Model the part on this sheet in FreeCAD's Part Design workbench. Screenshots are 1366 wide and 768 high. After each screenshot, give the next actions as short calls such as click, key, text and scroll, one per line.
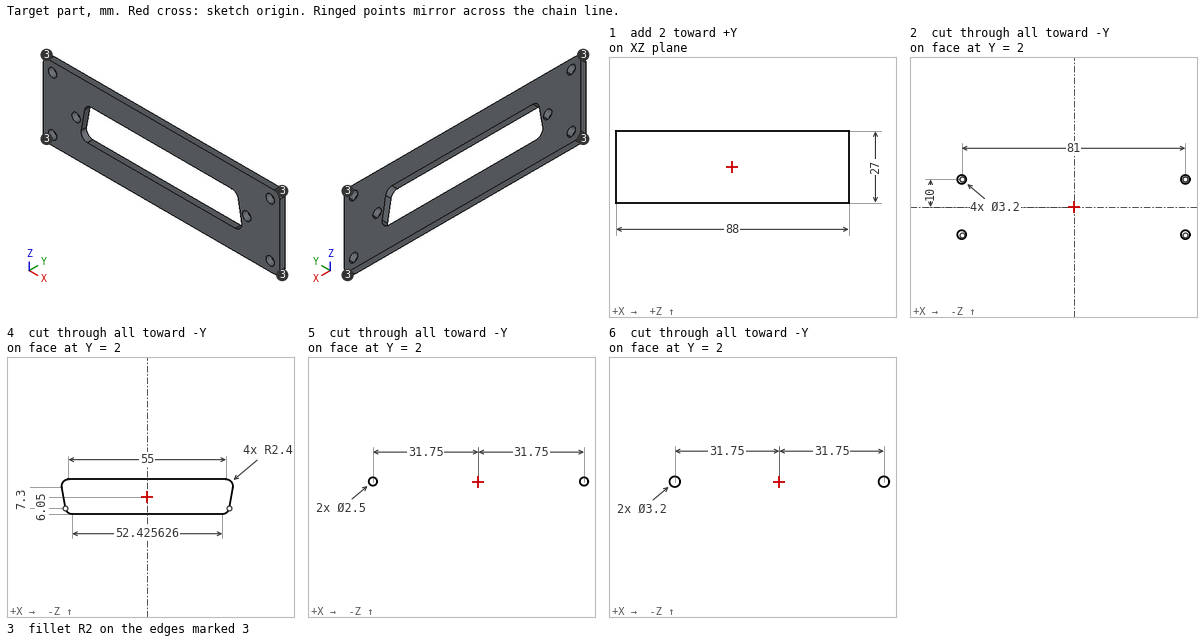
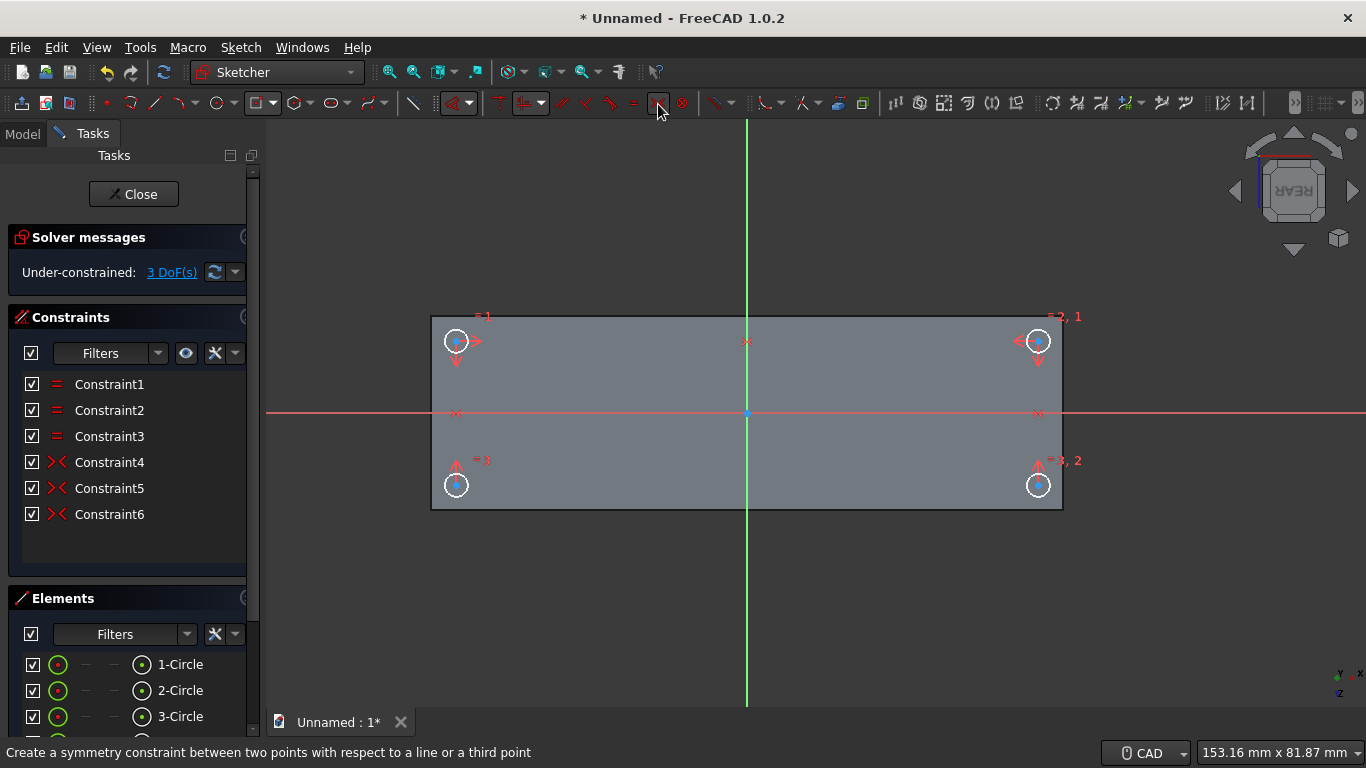
scroll(464, 333, up, 3)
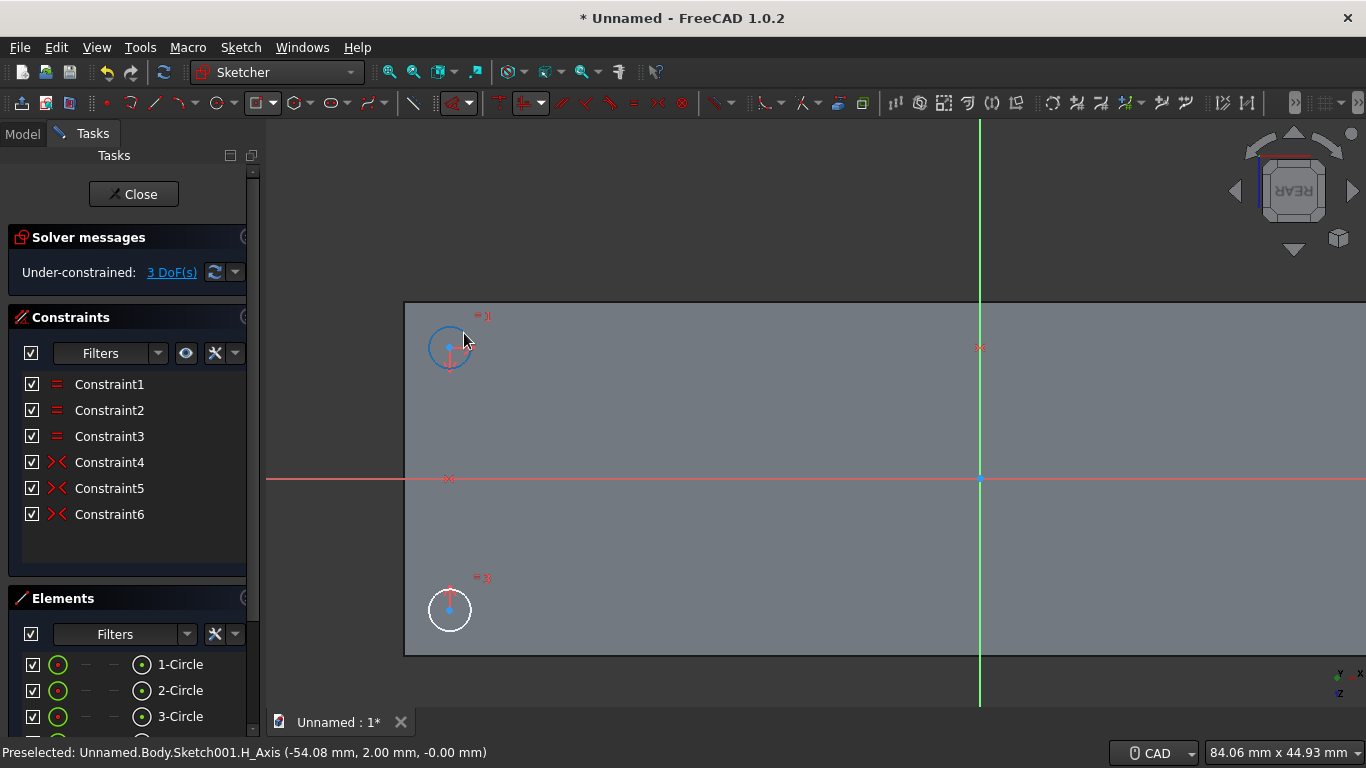
click(465, 333)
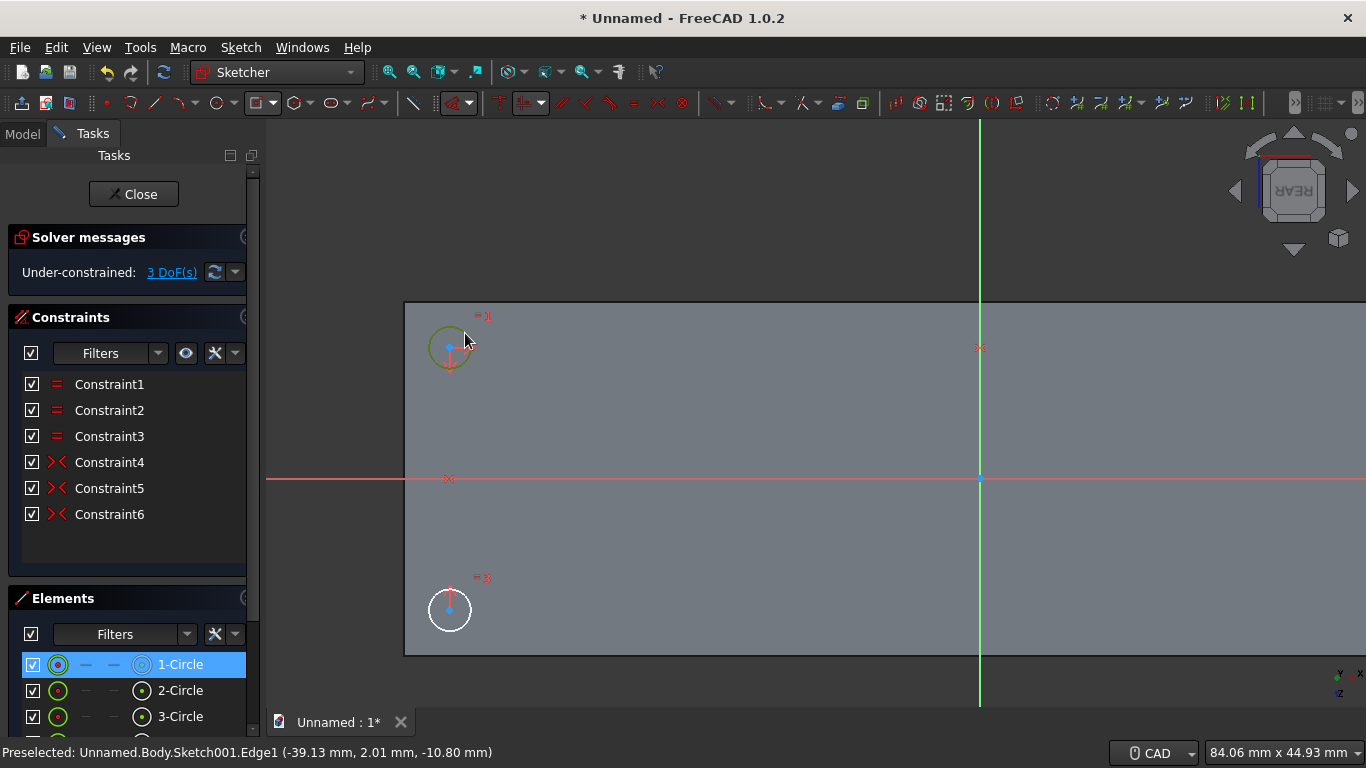
click(472, 104)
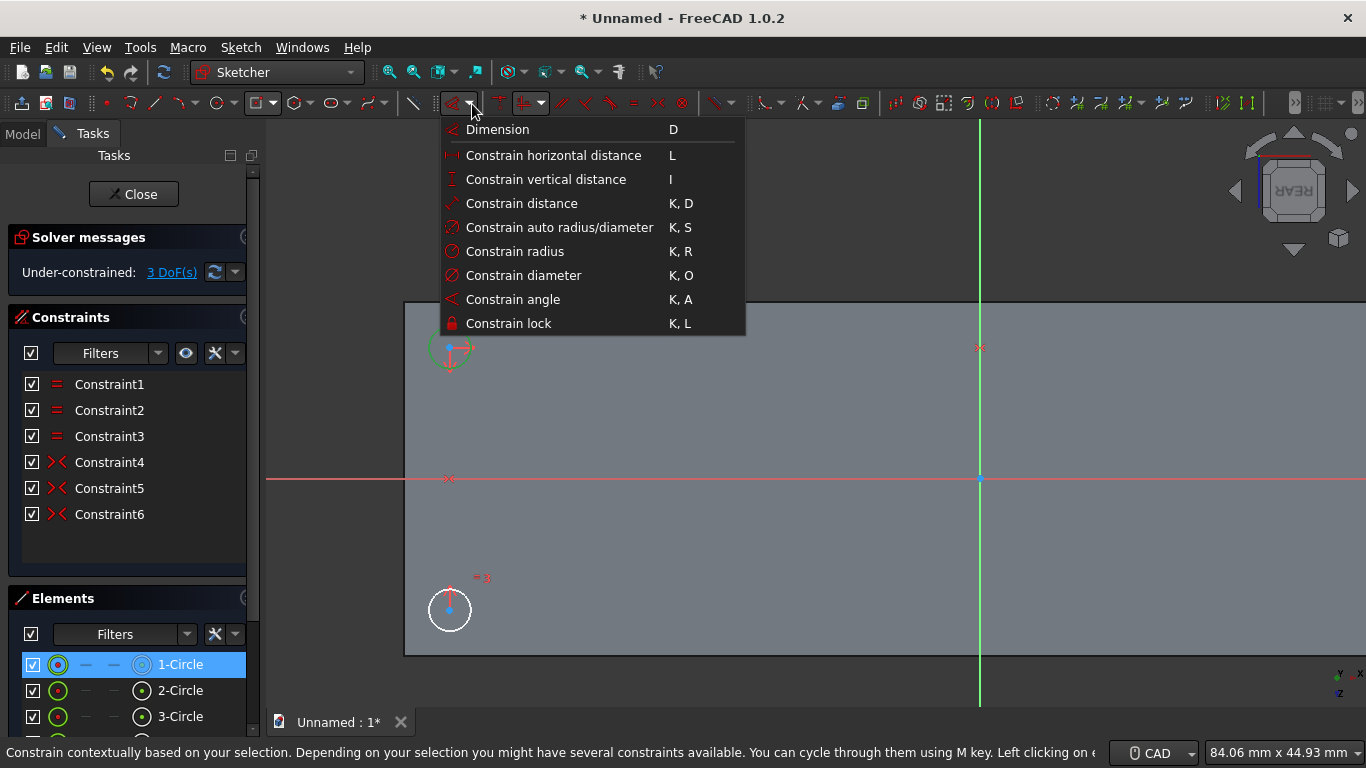
click(593, 275)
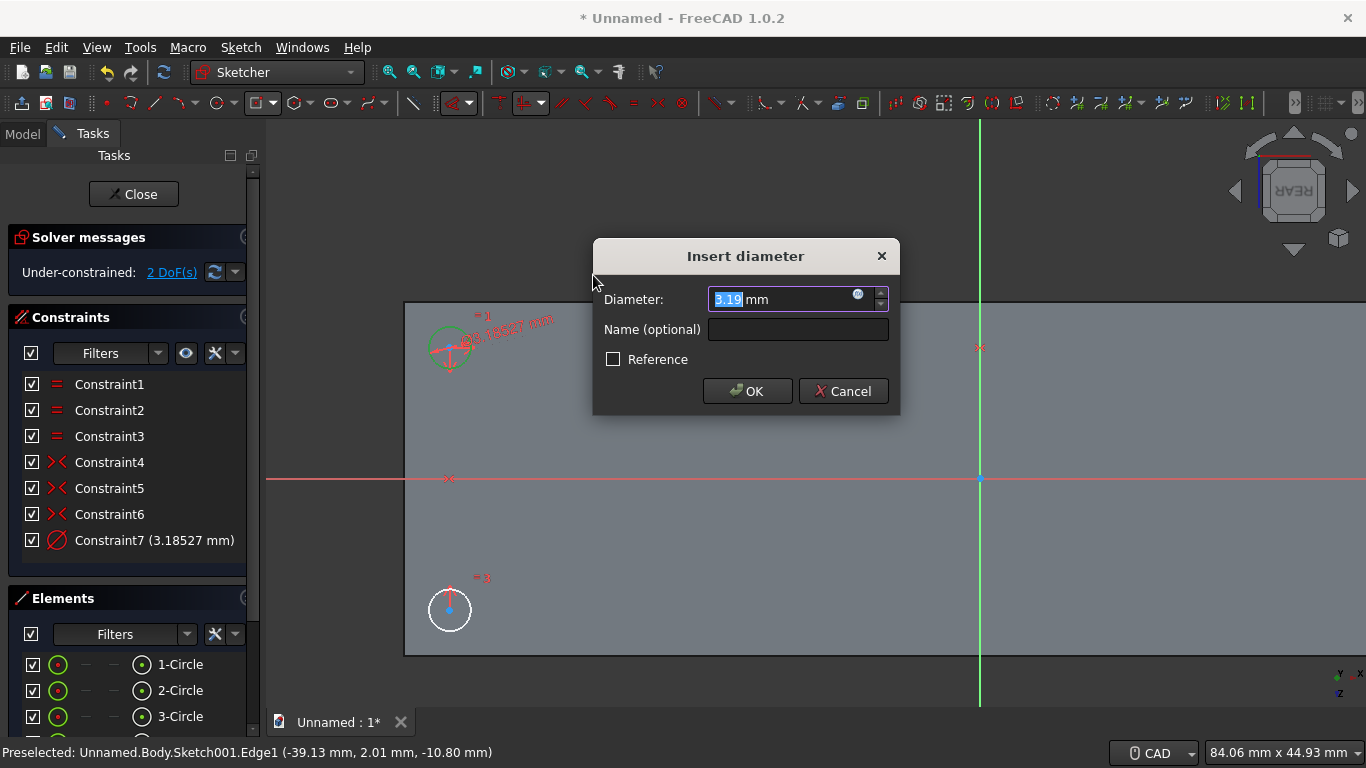
text(3.2)
key(Return)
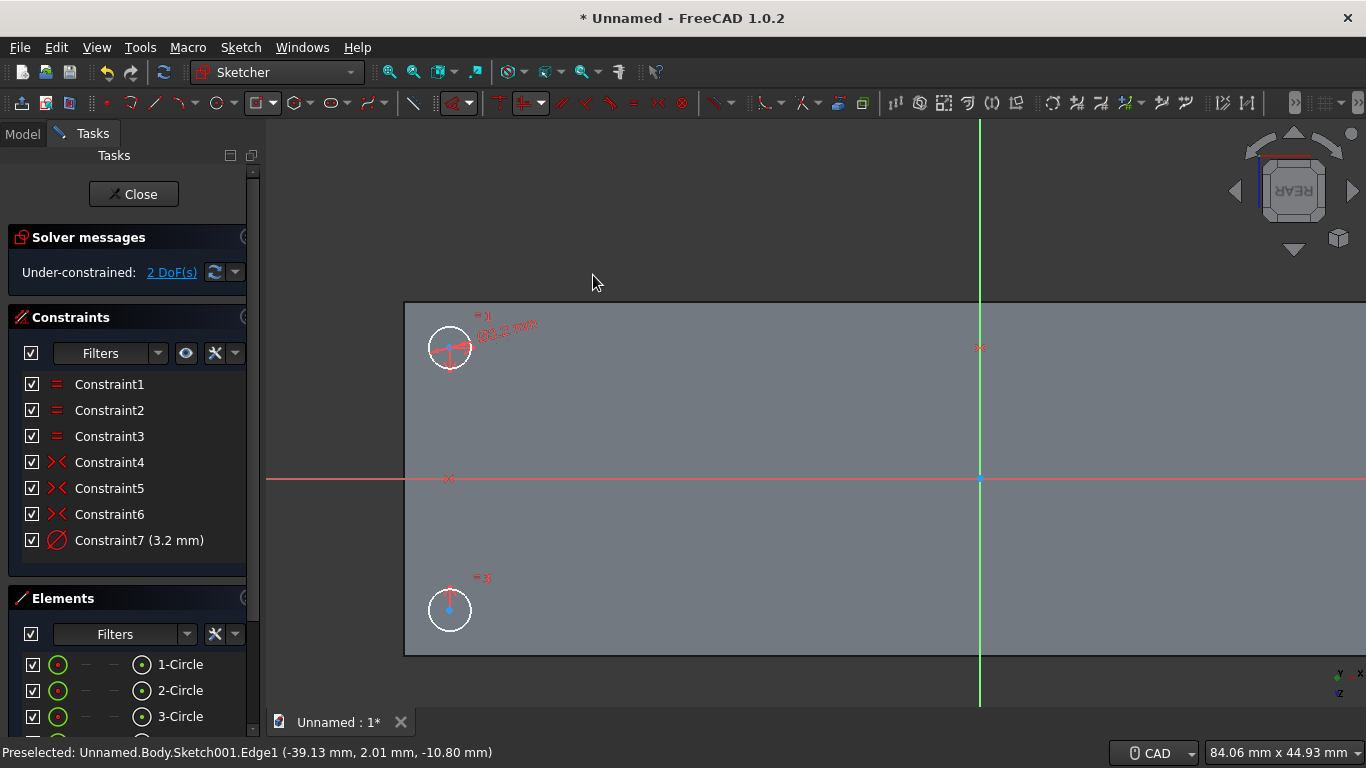
click(450, 348)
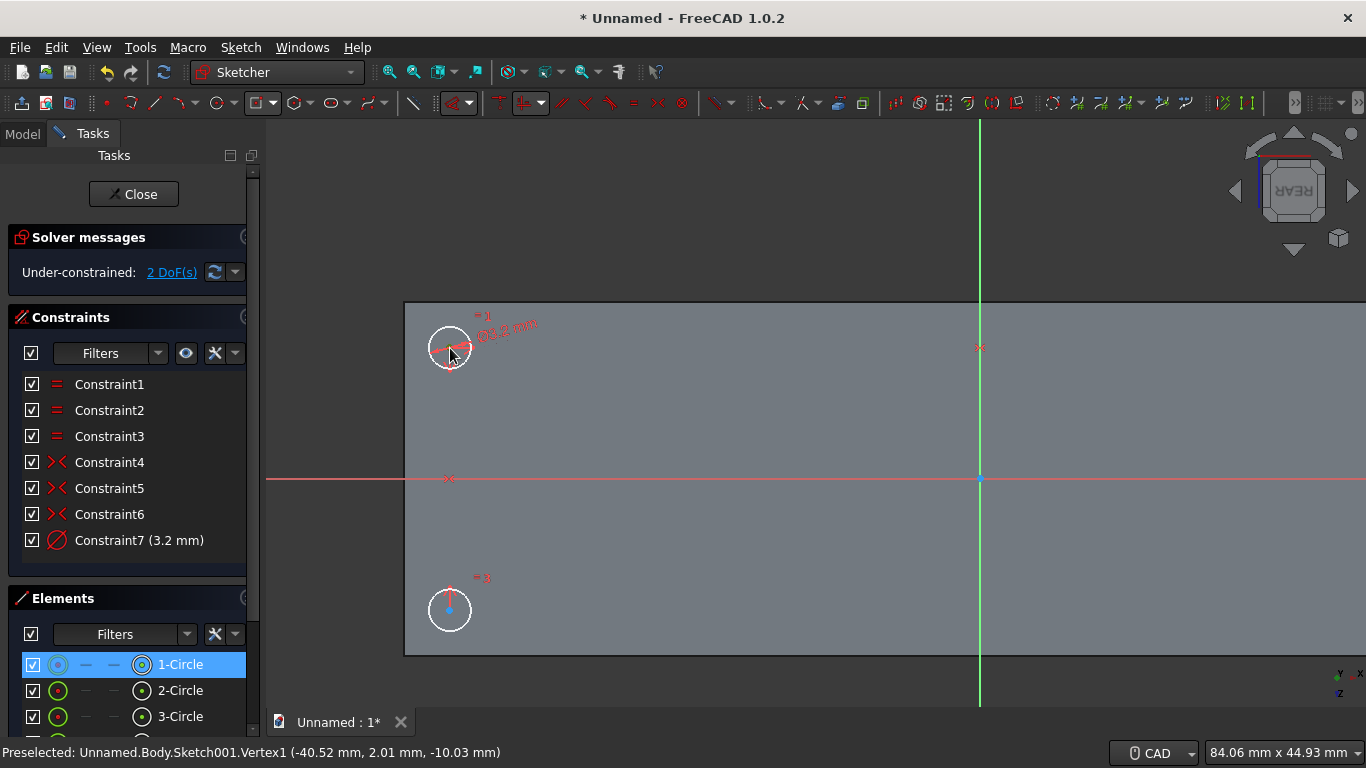
click(472, 104)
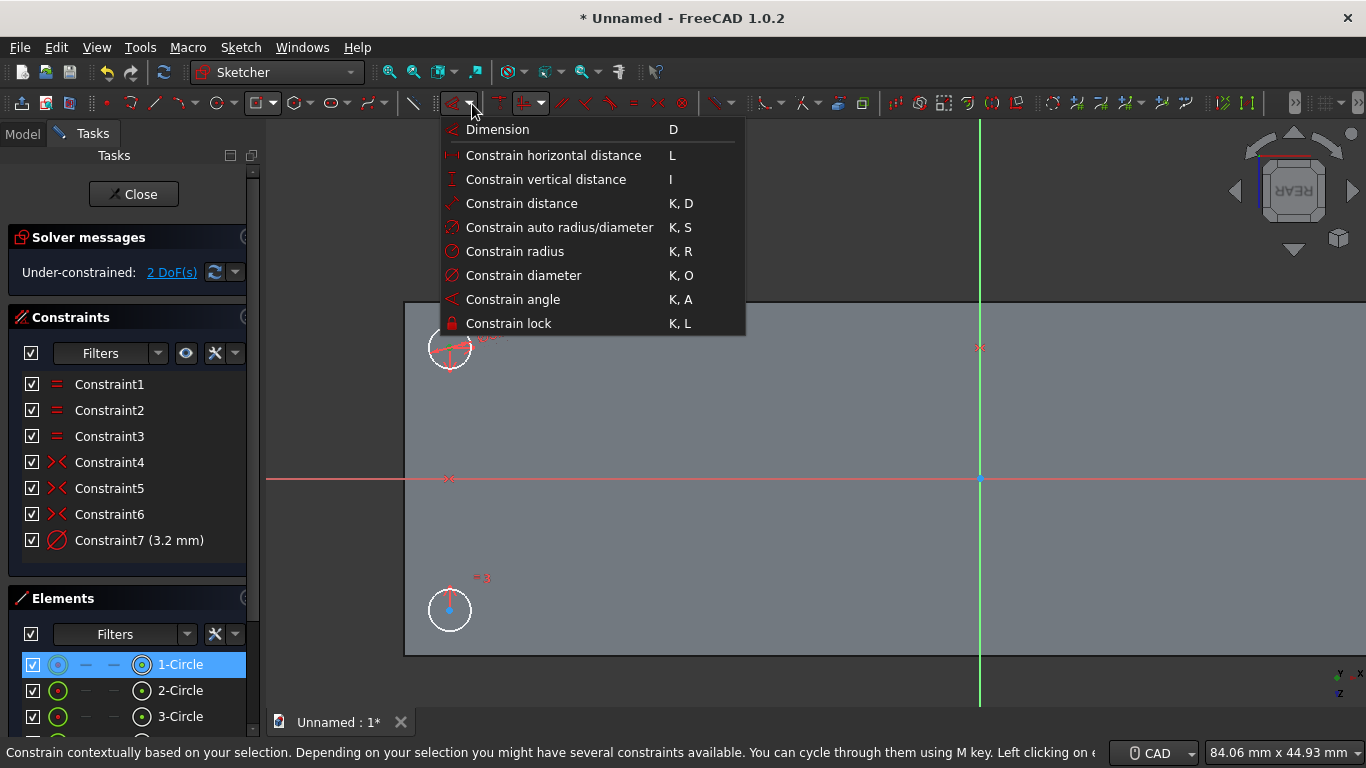
click(593, 179)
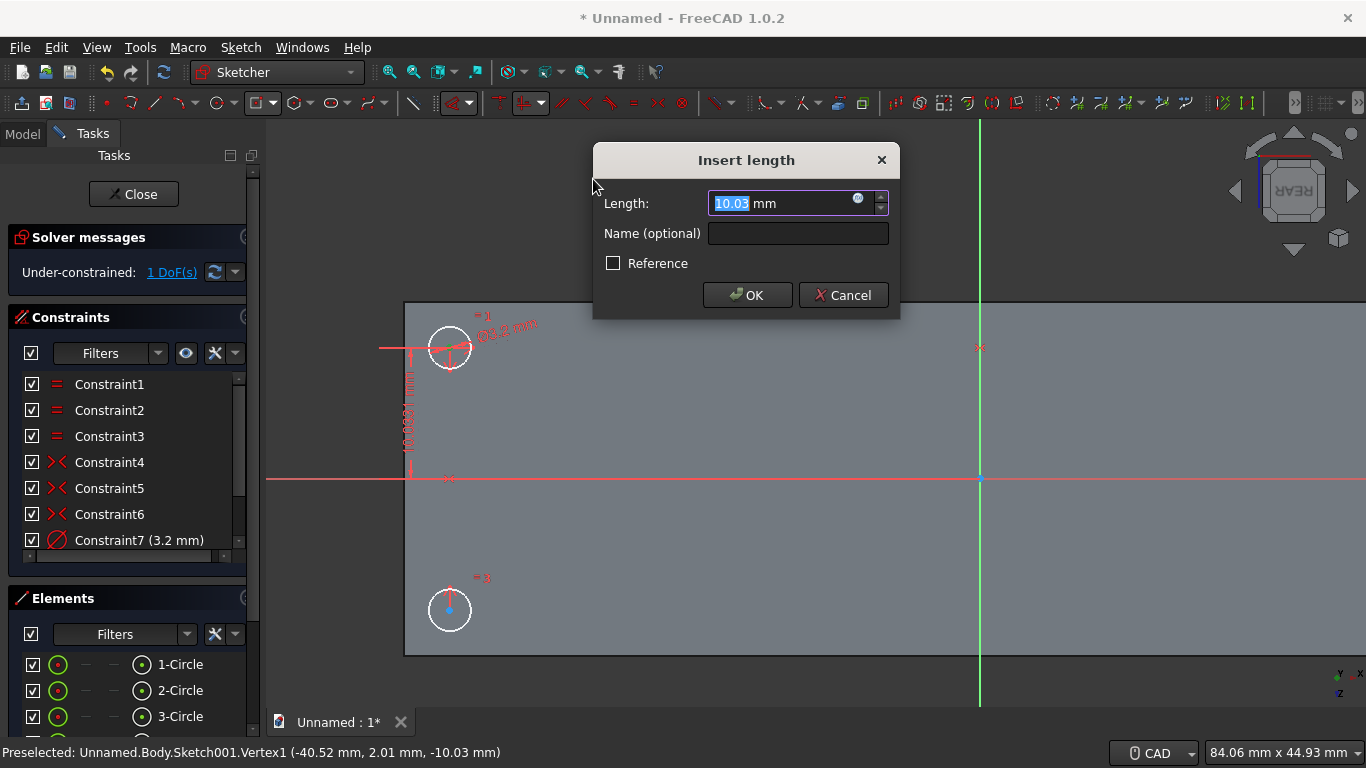
text(10)
key(Return)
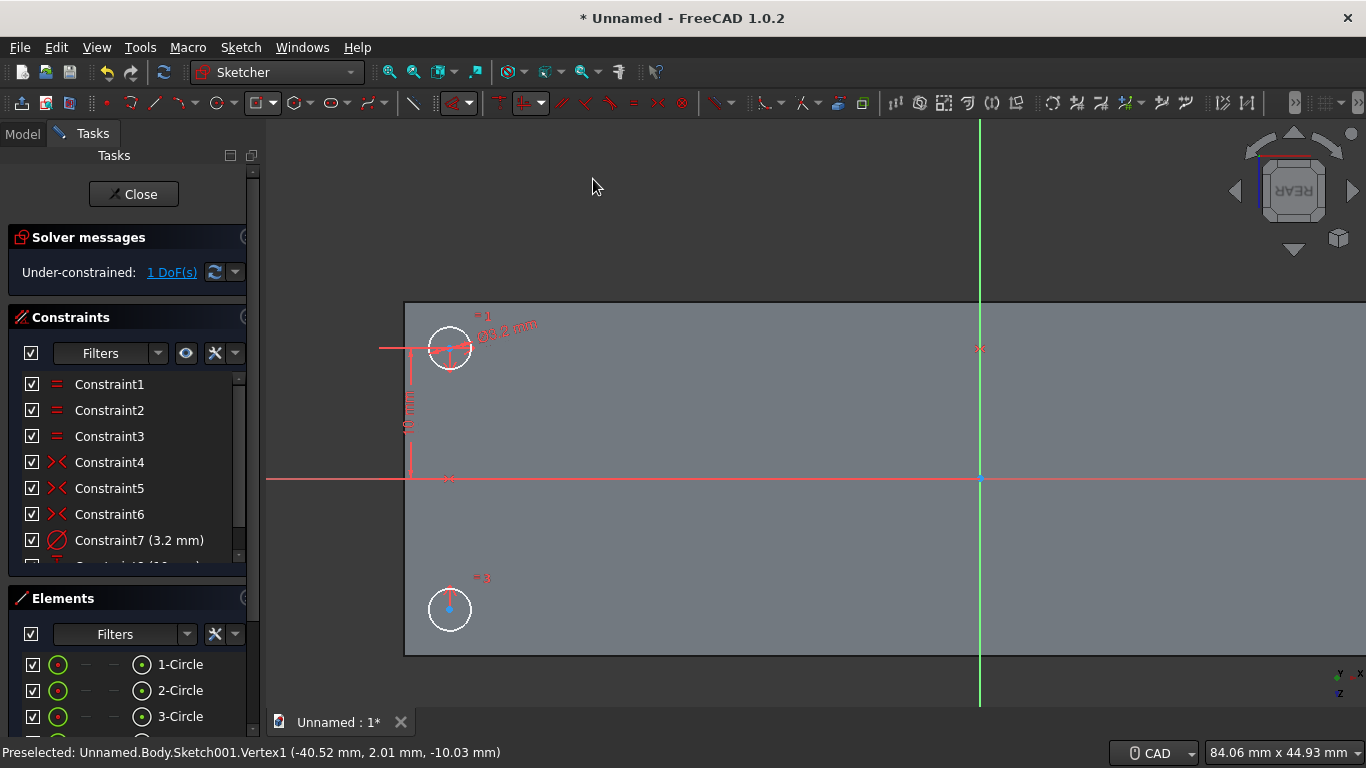
click(450, 348)